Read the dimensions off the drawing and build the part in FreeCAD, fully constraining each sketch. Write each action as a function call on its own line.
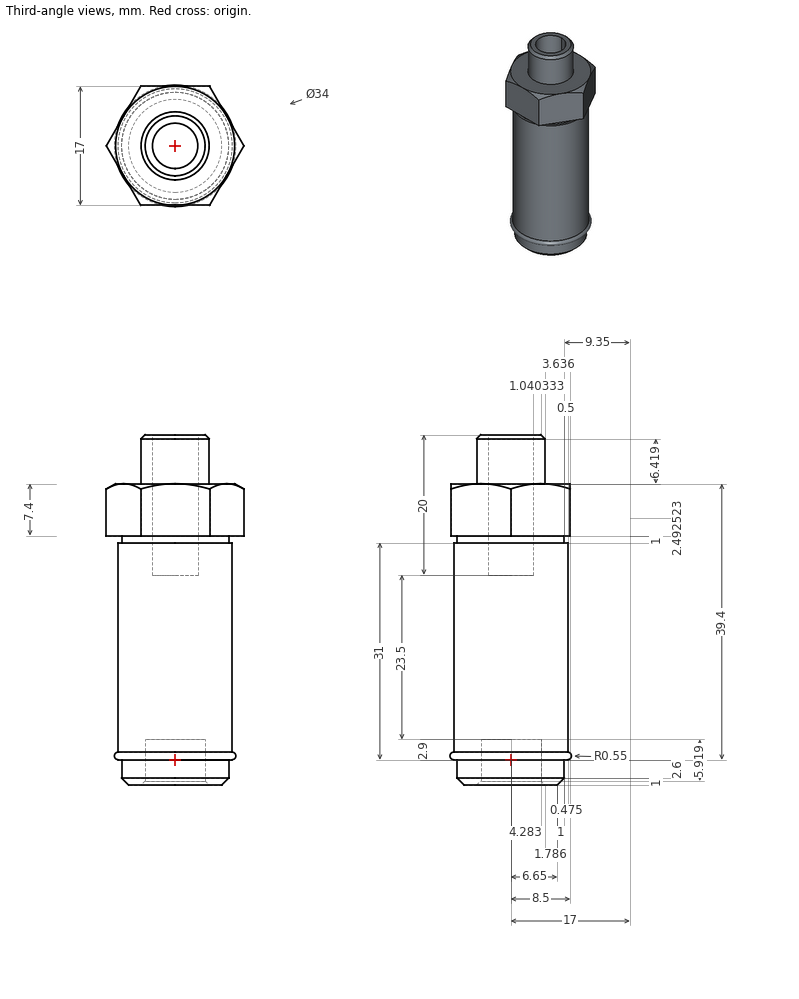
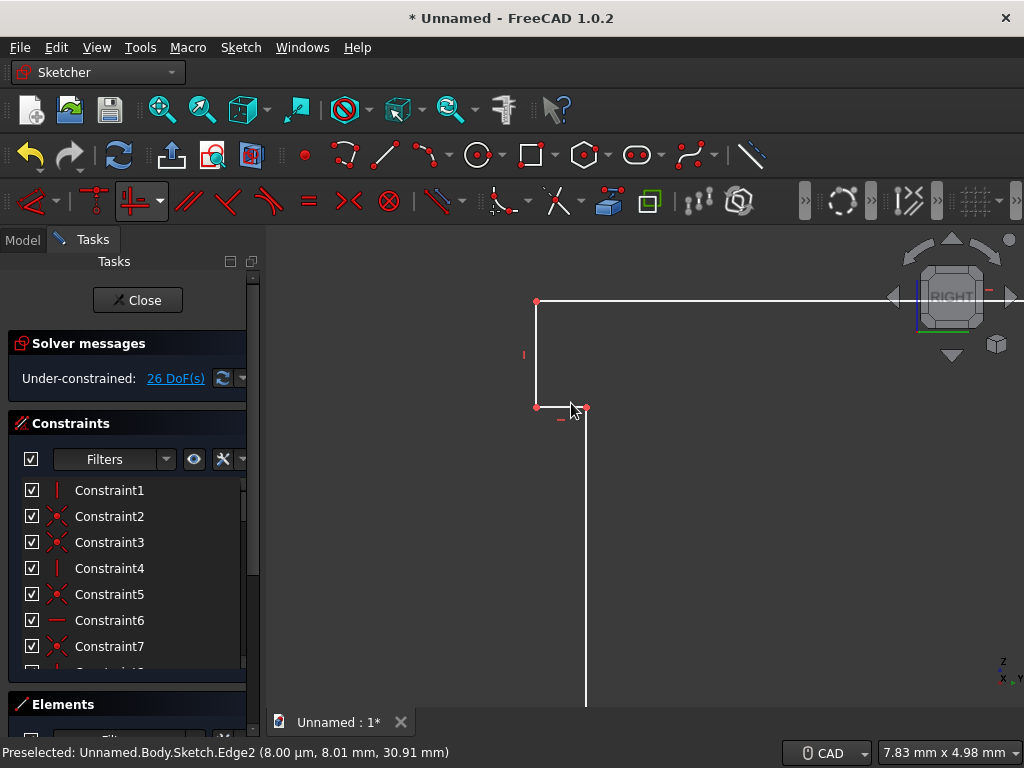
scroll(574, 410, down, 14)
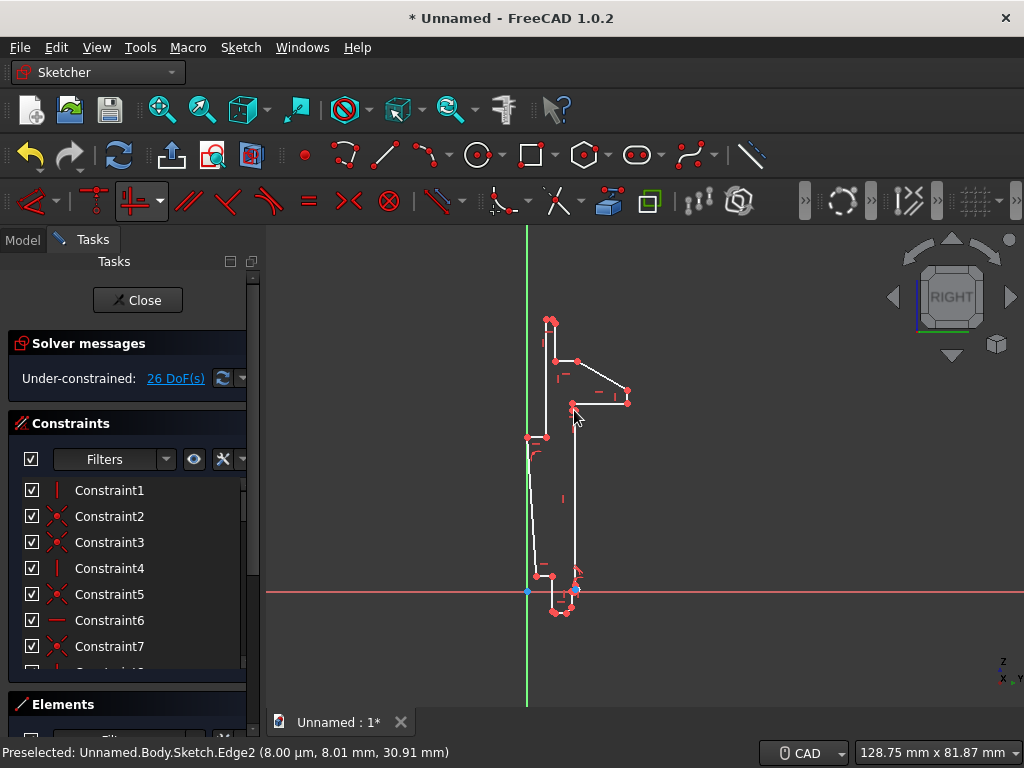
scroll(530, 479, up, 9)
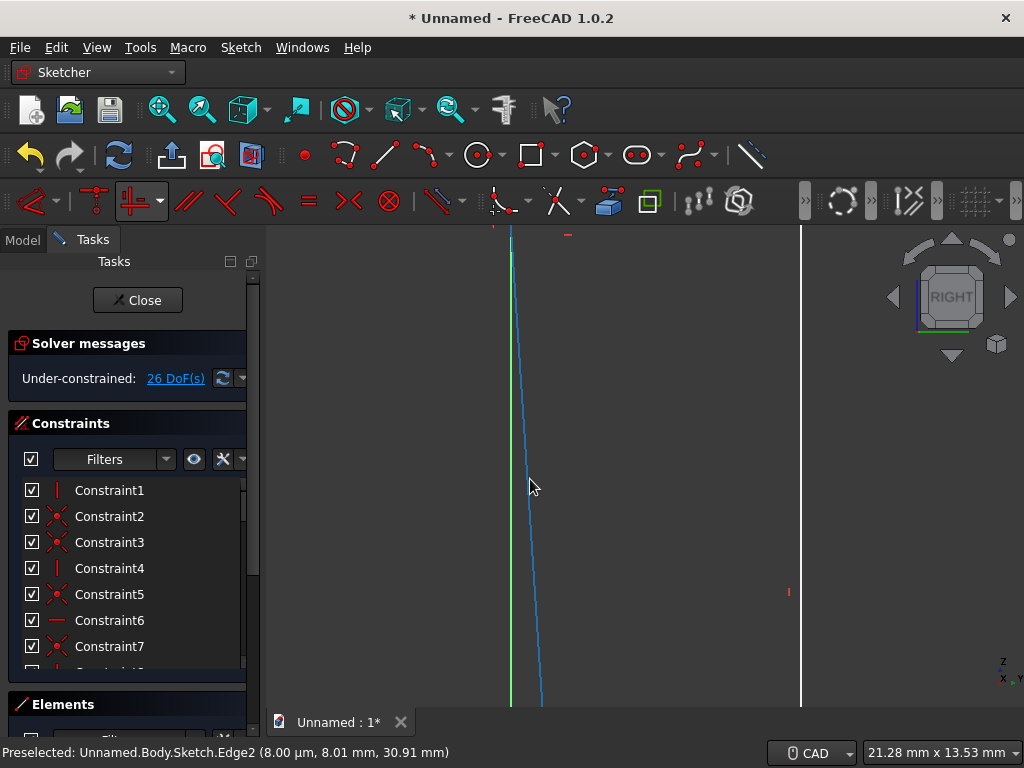
click(527, 475)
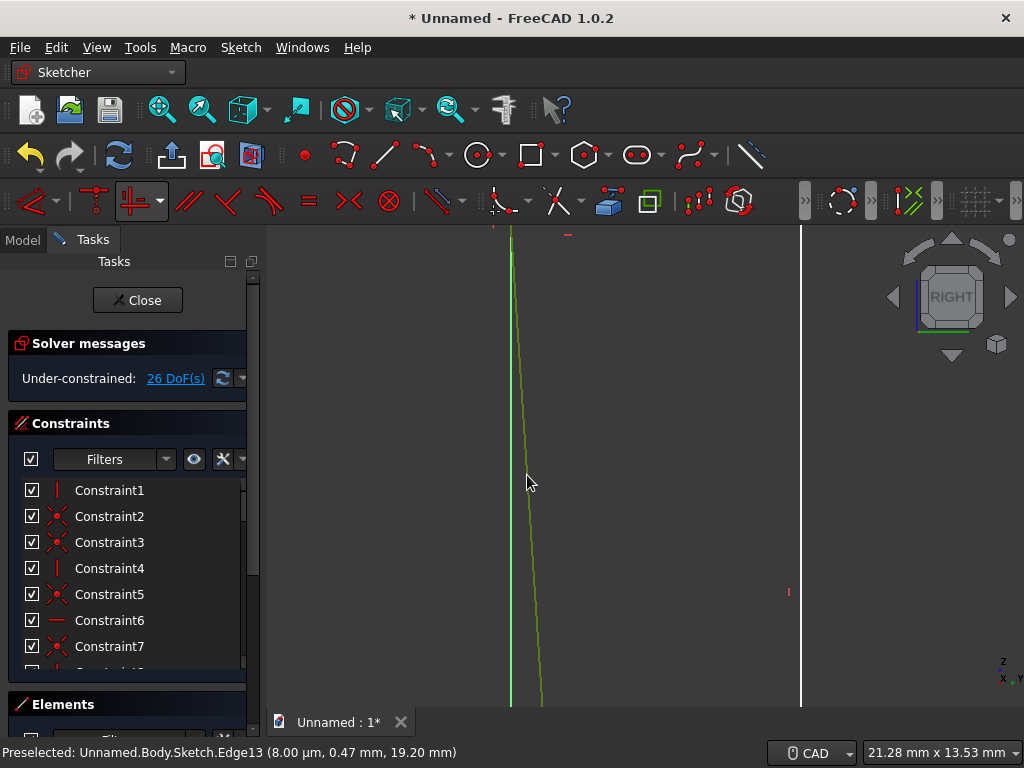
key(v)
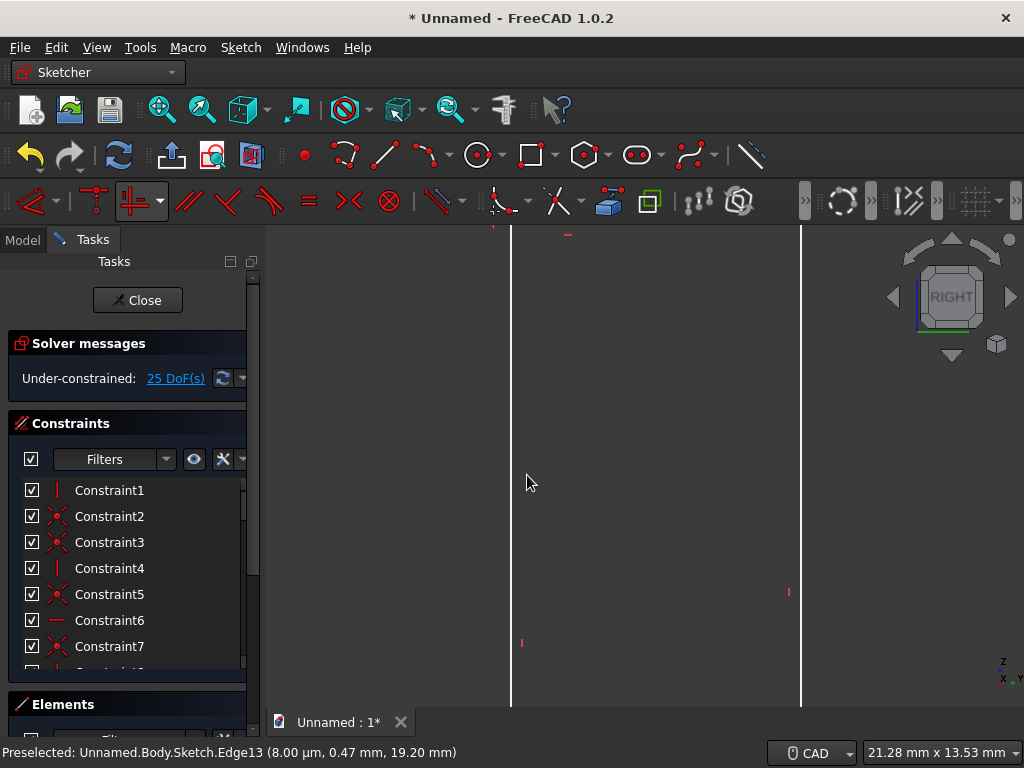
scroll(530, 480, down, 9)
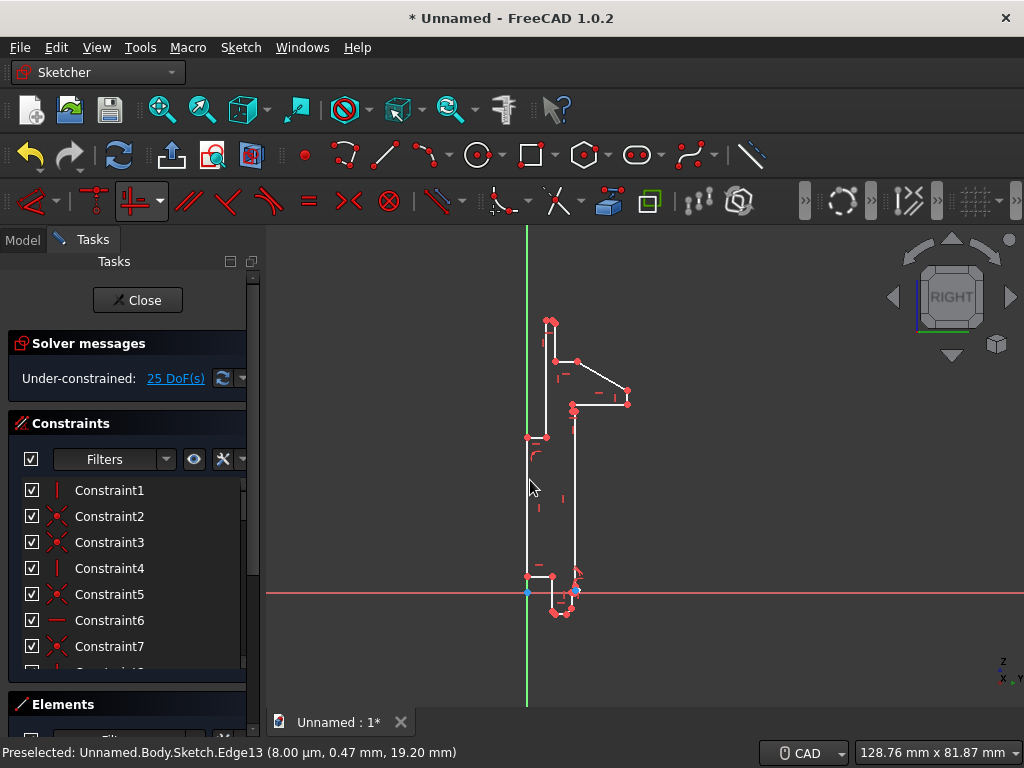
scroll(573, 593, up, 12)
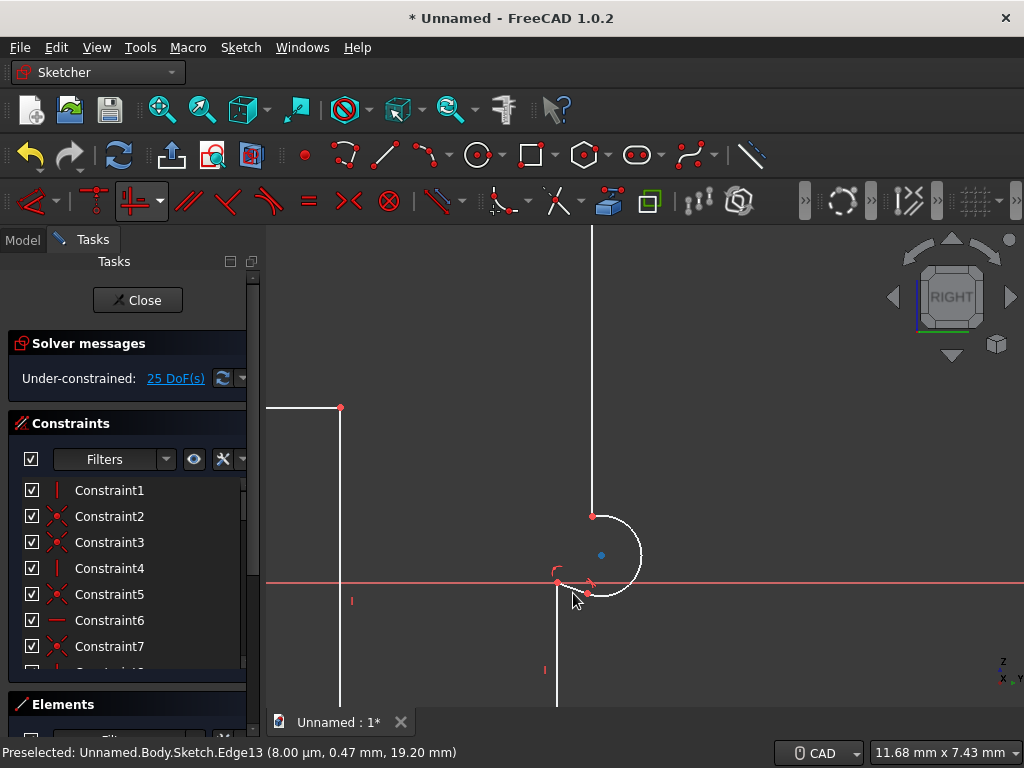
click(573, 588)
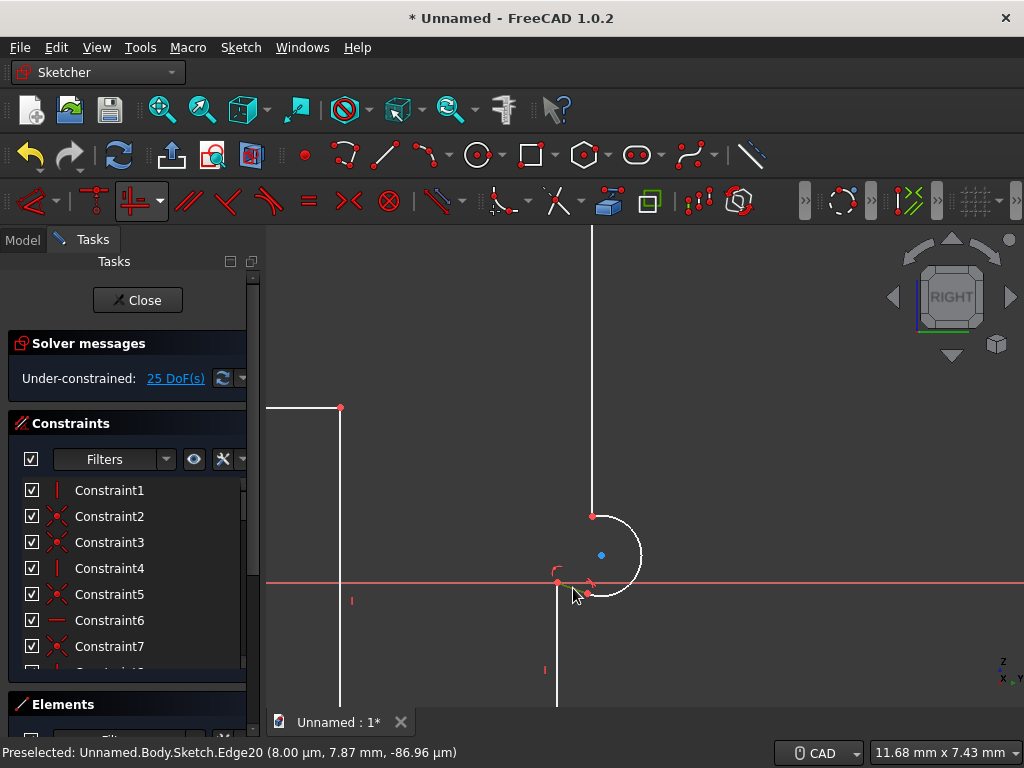
key(h)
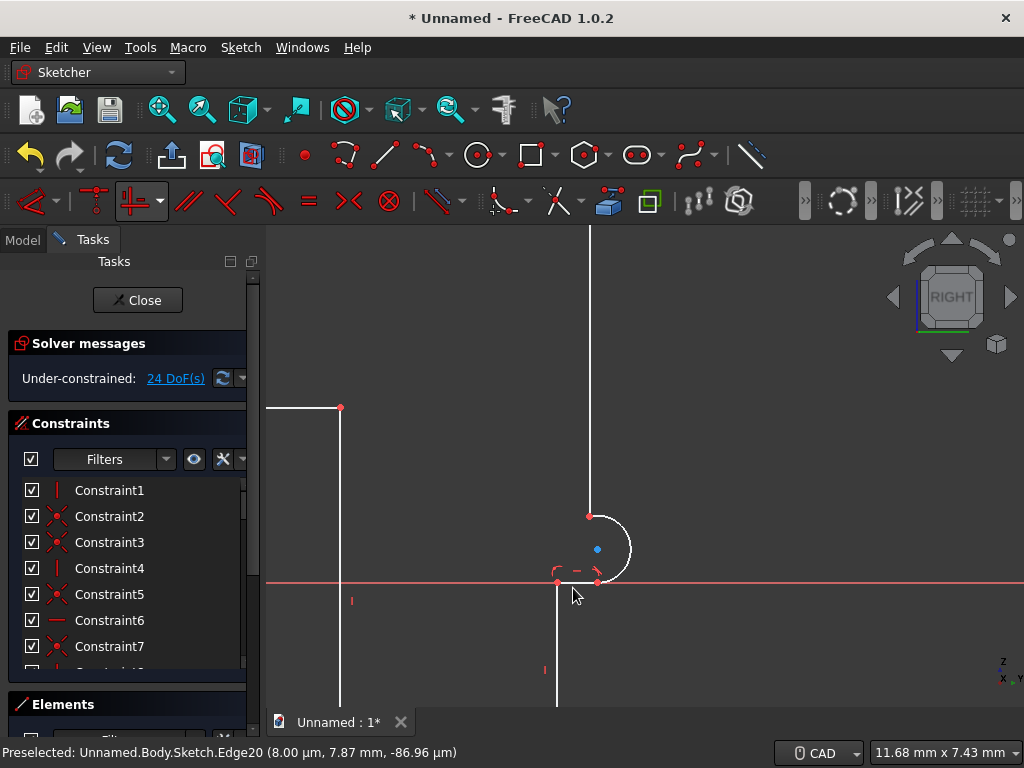
click(626, 567)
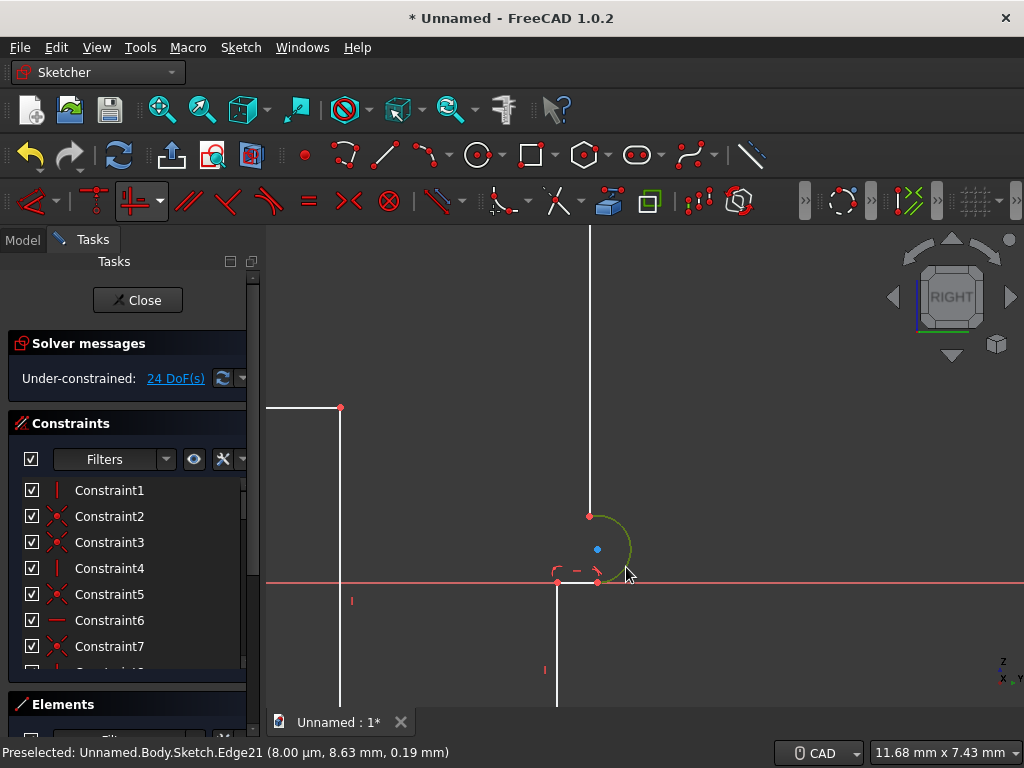
key(k)
key(r)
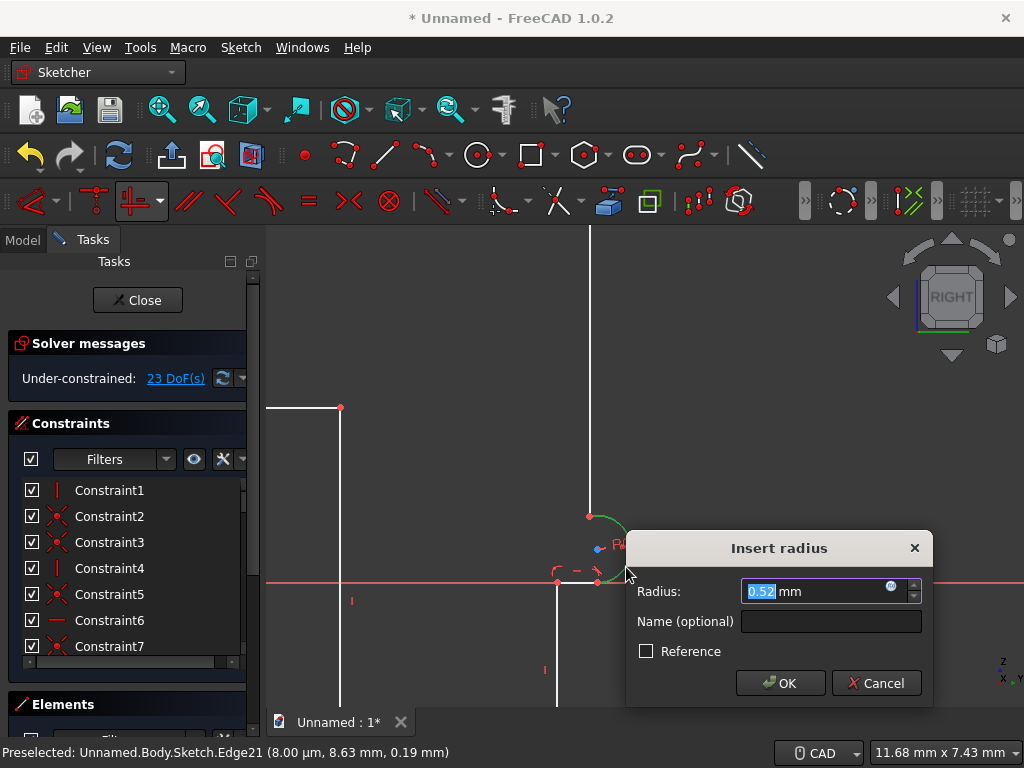
text(0.55)
key(Return)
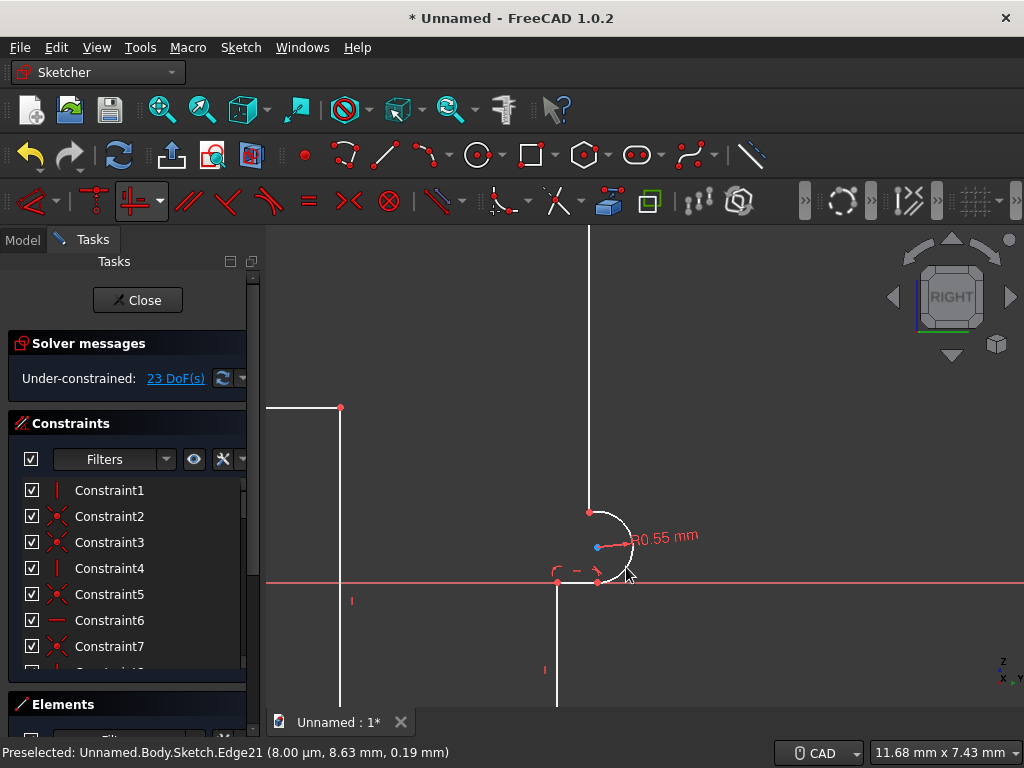
scroll(573, 593, down, 12)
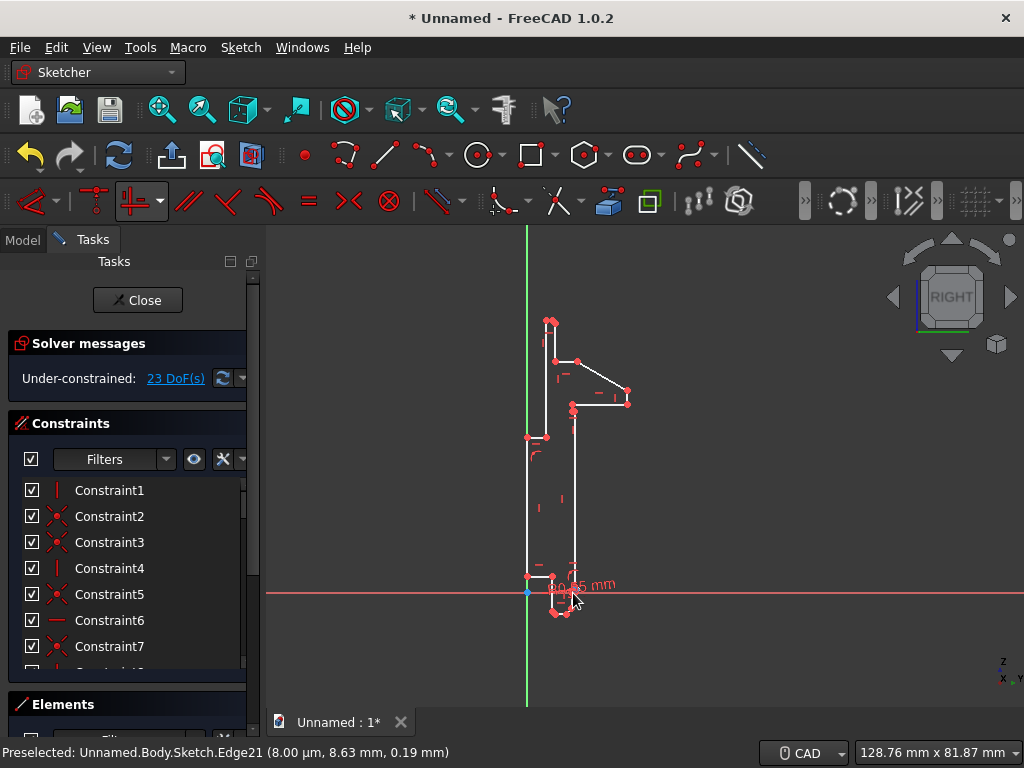
scroll(572, 409, up, 10)